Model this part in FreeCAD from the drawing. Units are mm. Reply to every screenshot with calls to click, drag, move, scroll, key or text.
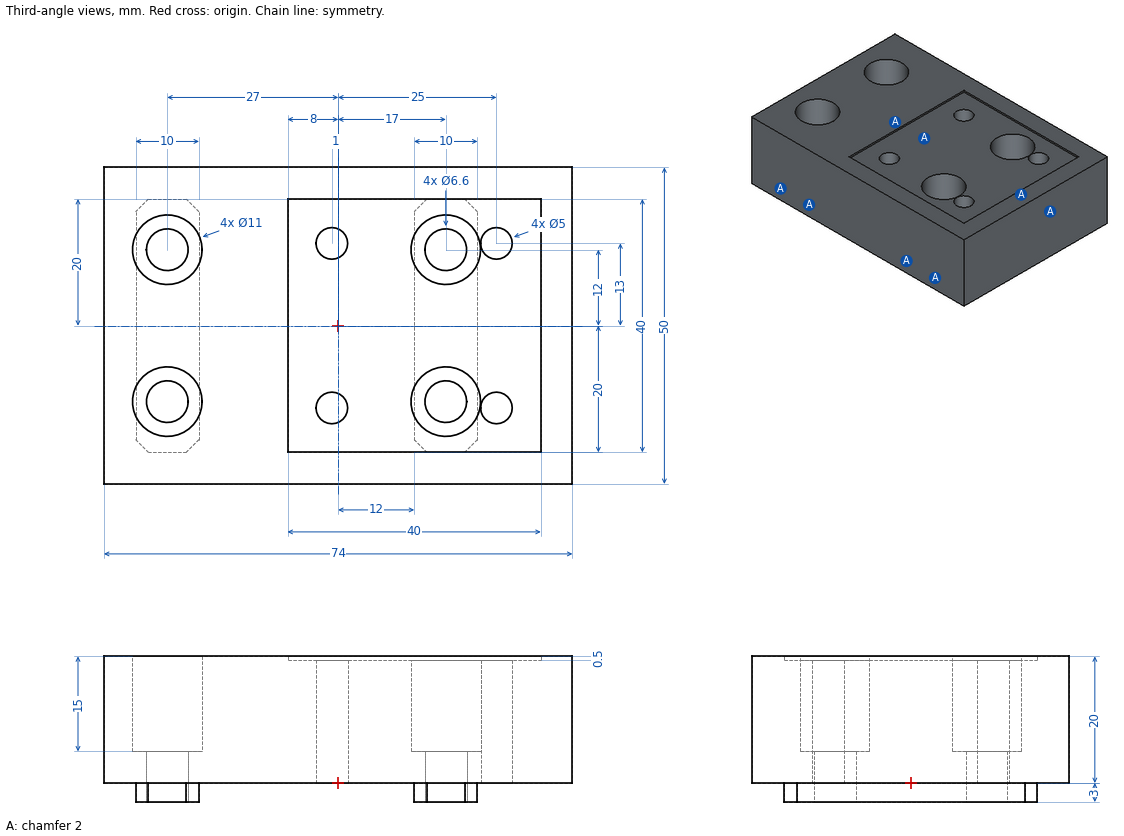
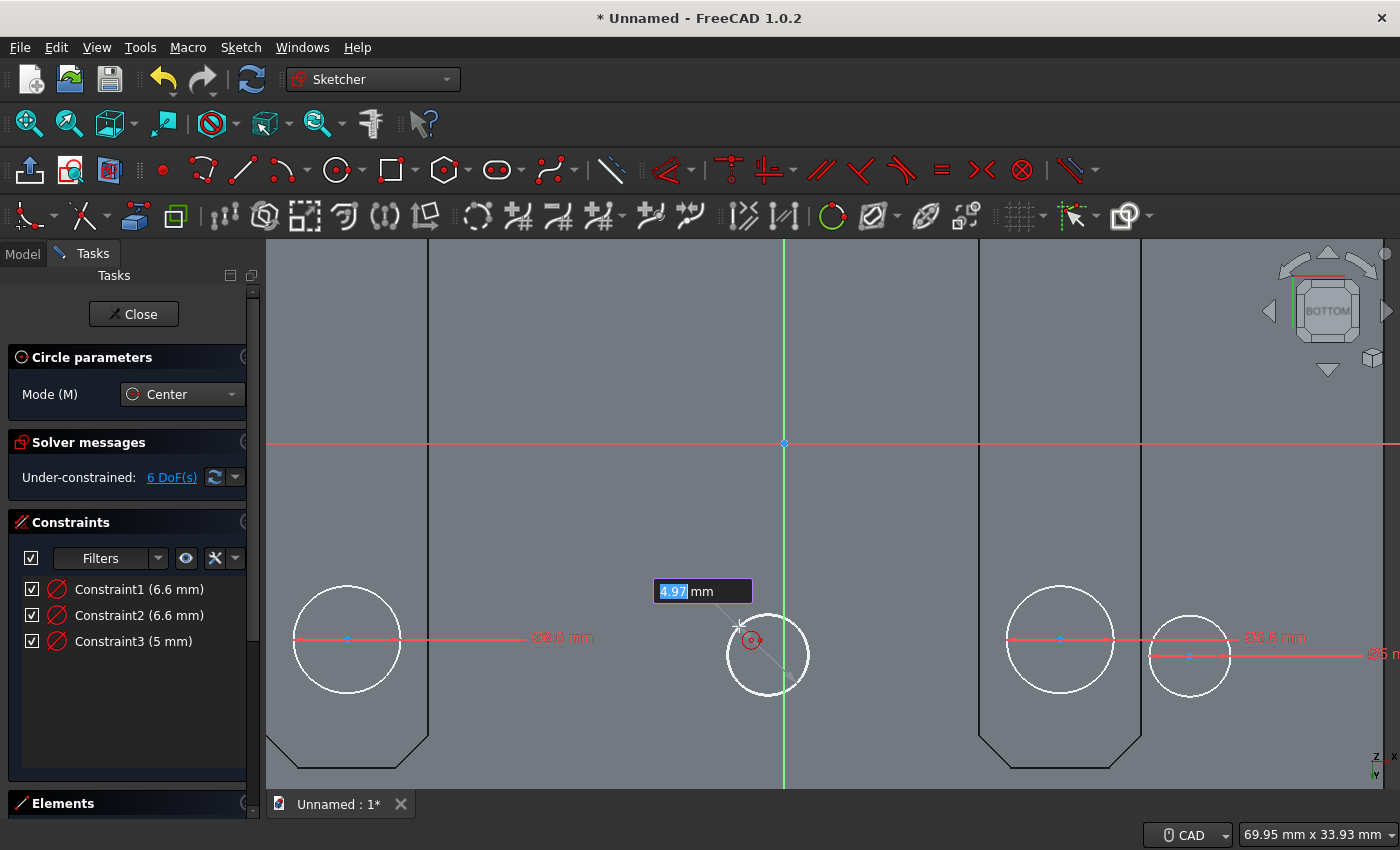
text(5)
key(Return)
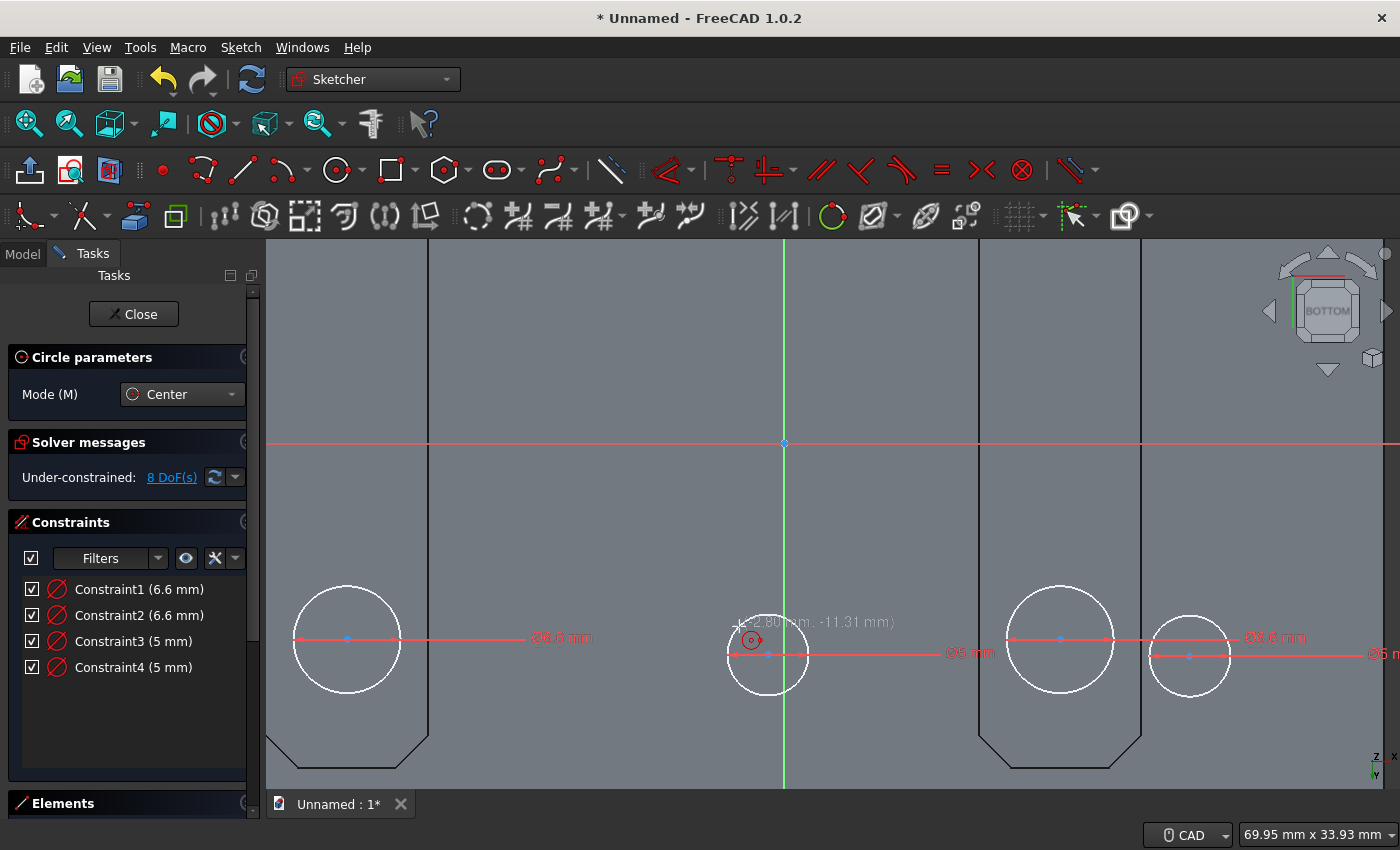
scroll(770, 657, down, 2)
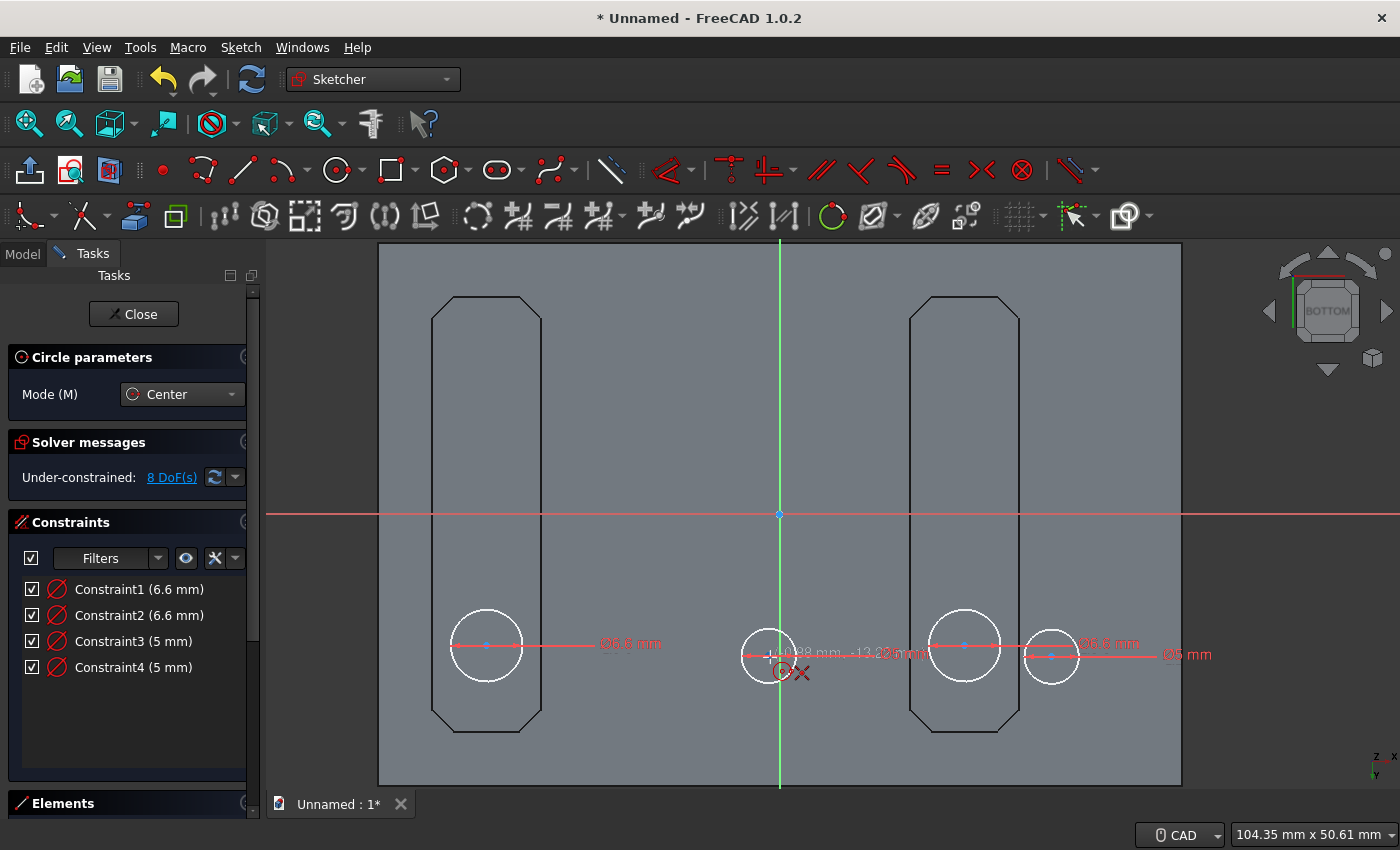
scroll(769, 373, up, 2)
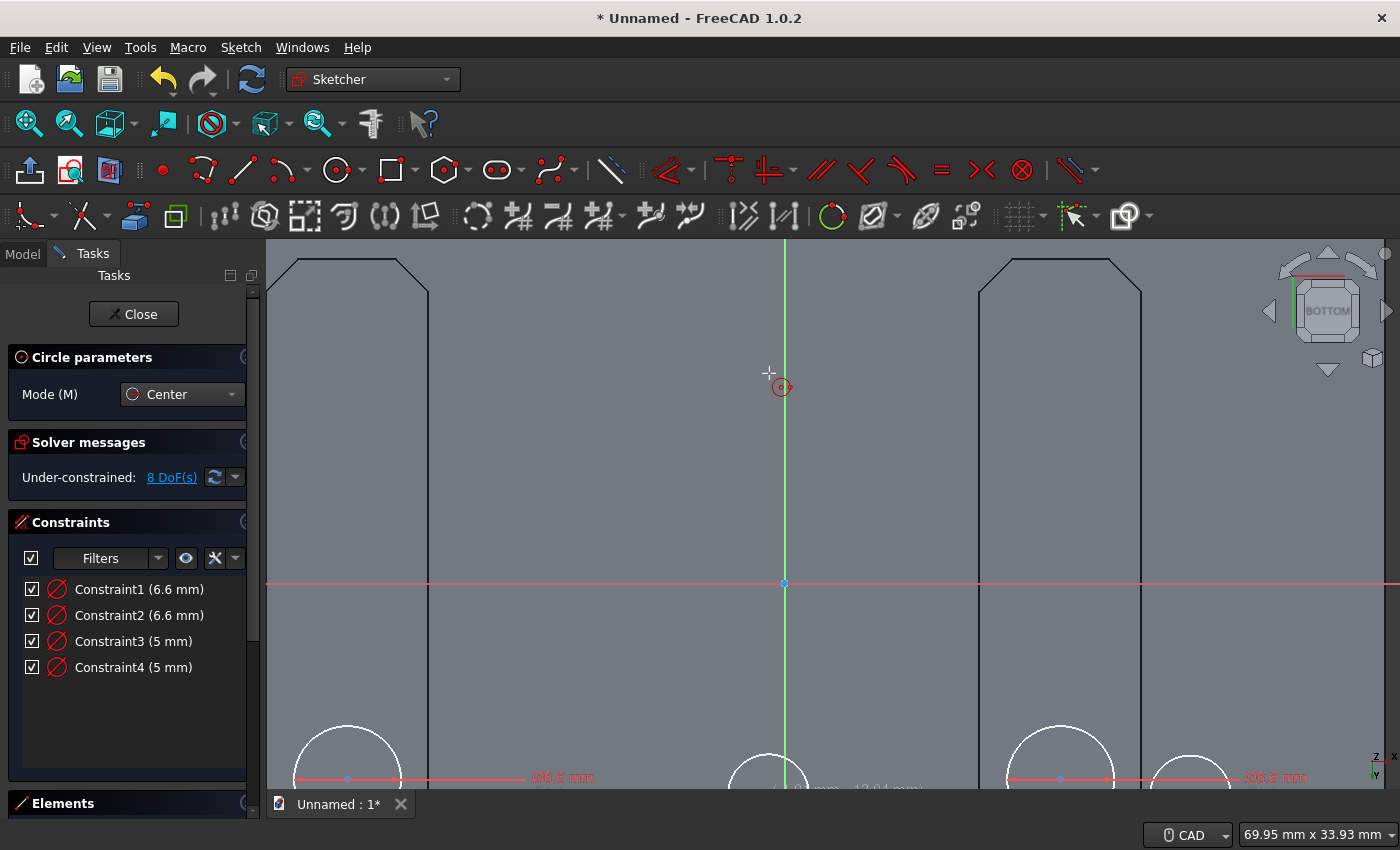
click(769, 373)
move(740, 344)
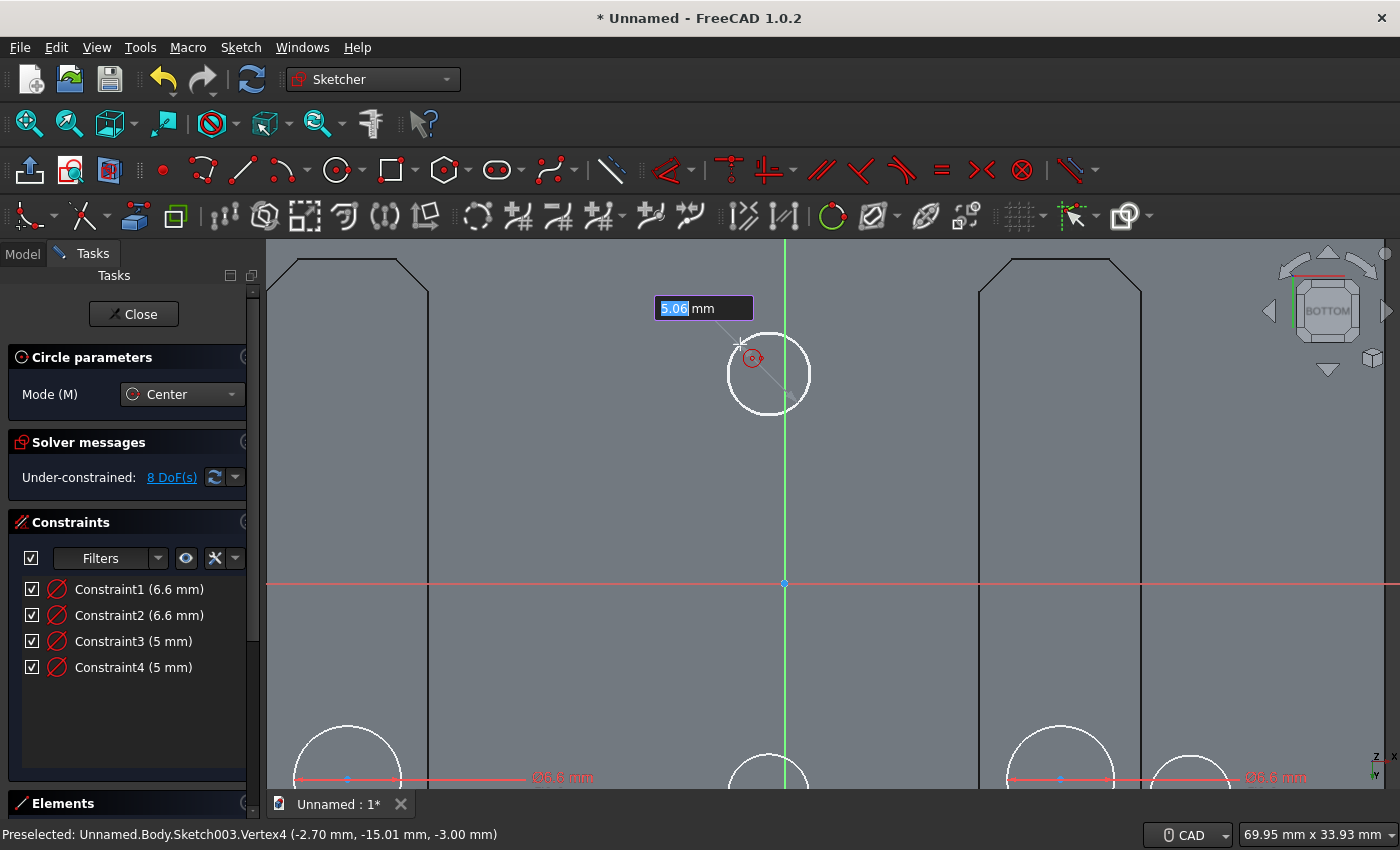
text(5)
key(Return)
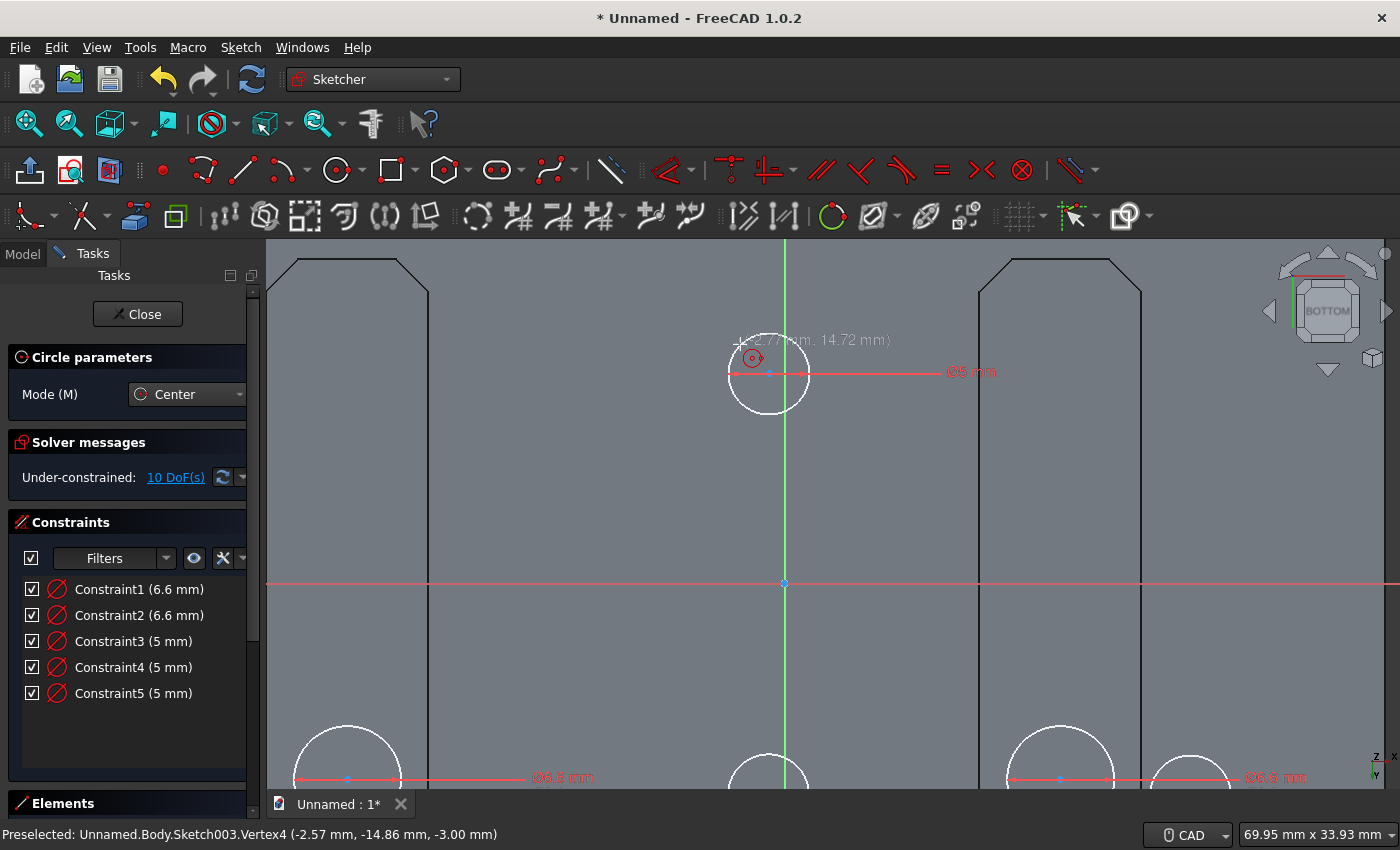
click(1190, 373)
move(1219, 344)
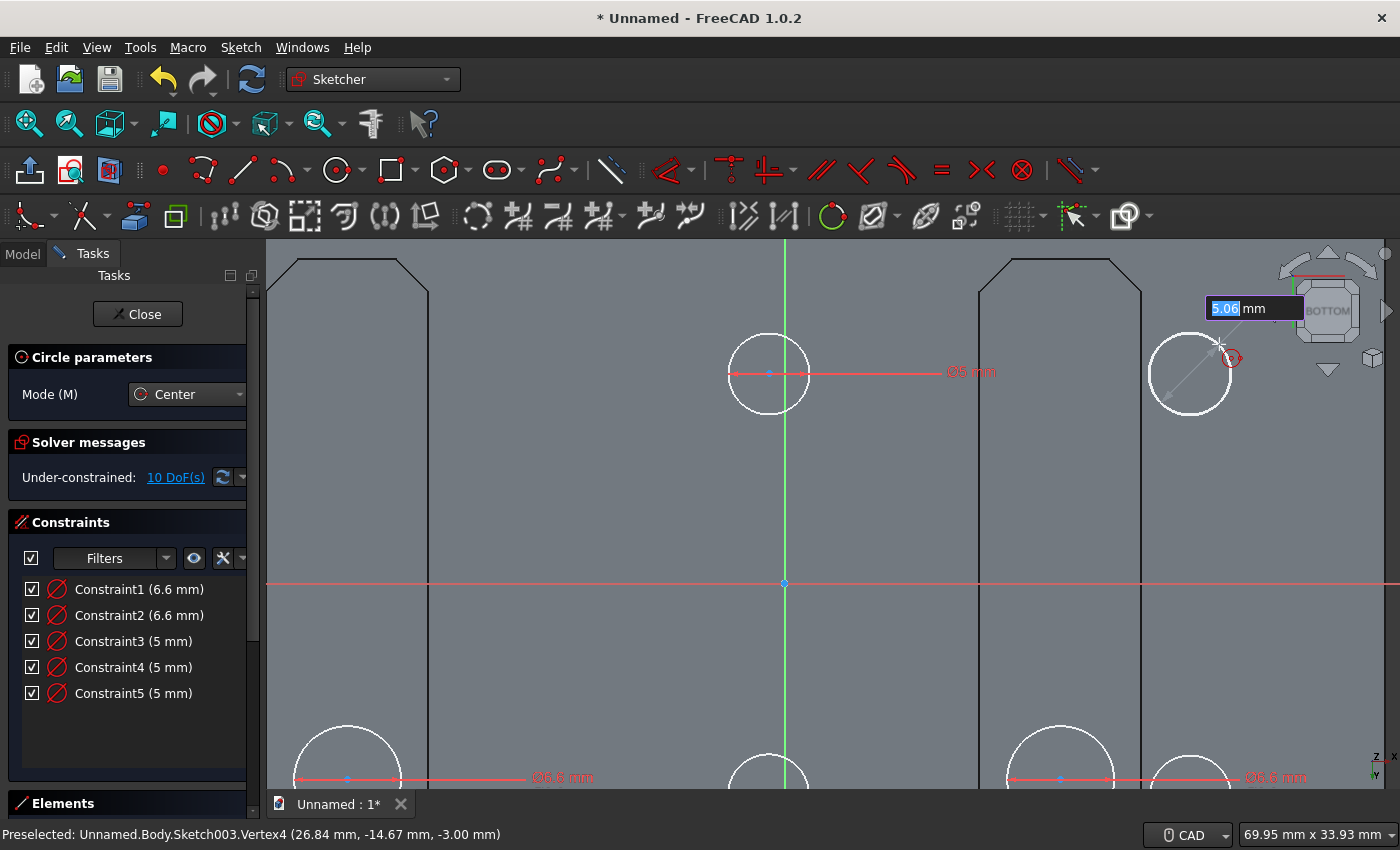
text(5)
key(Return)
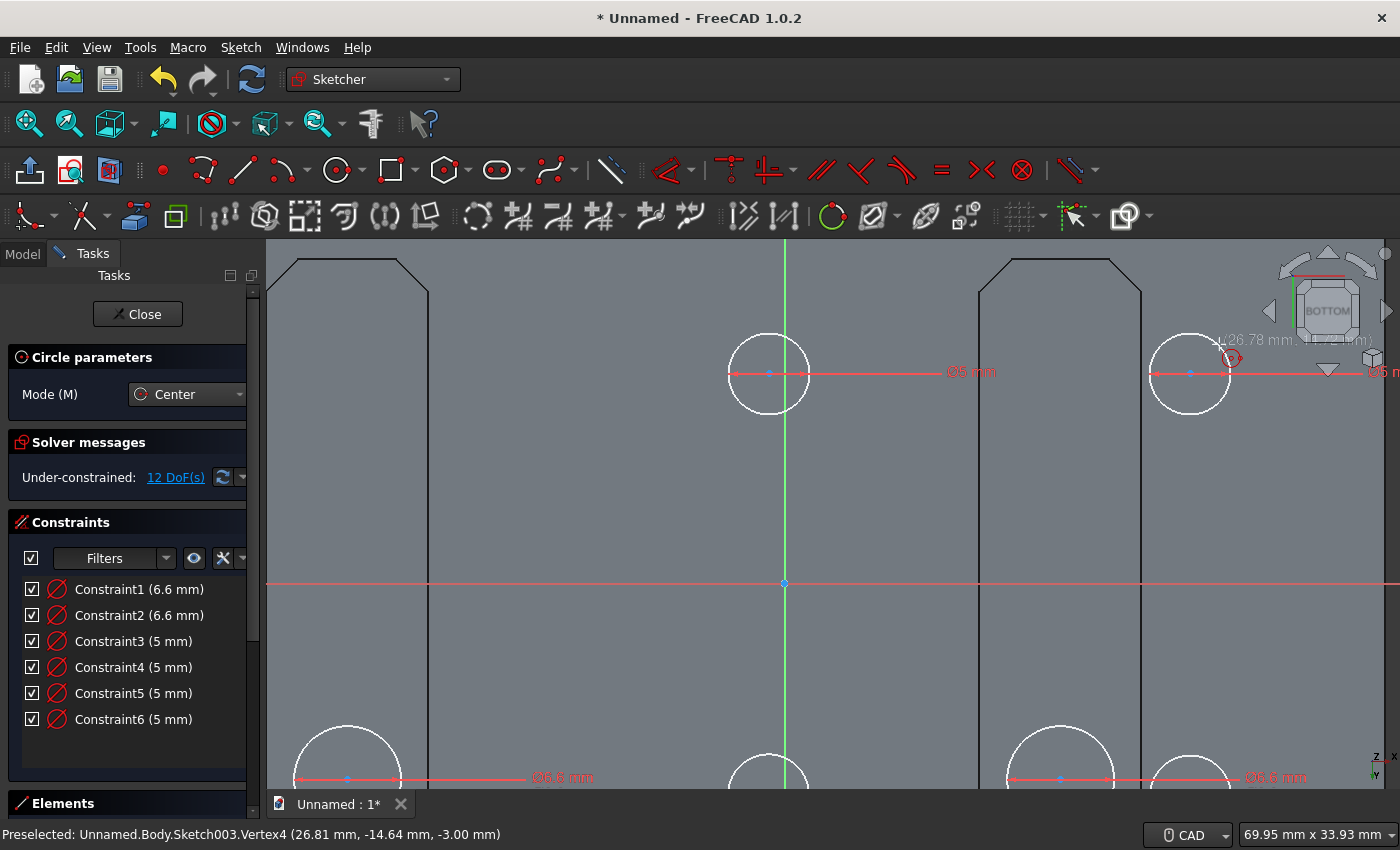
click(347, 389)
move(385, 351)